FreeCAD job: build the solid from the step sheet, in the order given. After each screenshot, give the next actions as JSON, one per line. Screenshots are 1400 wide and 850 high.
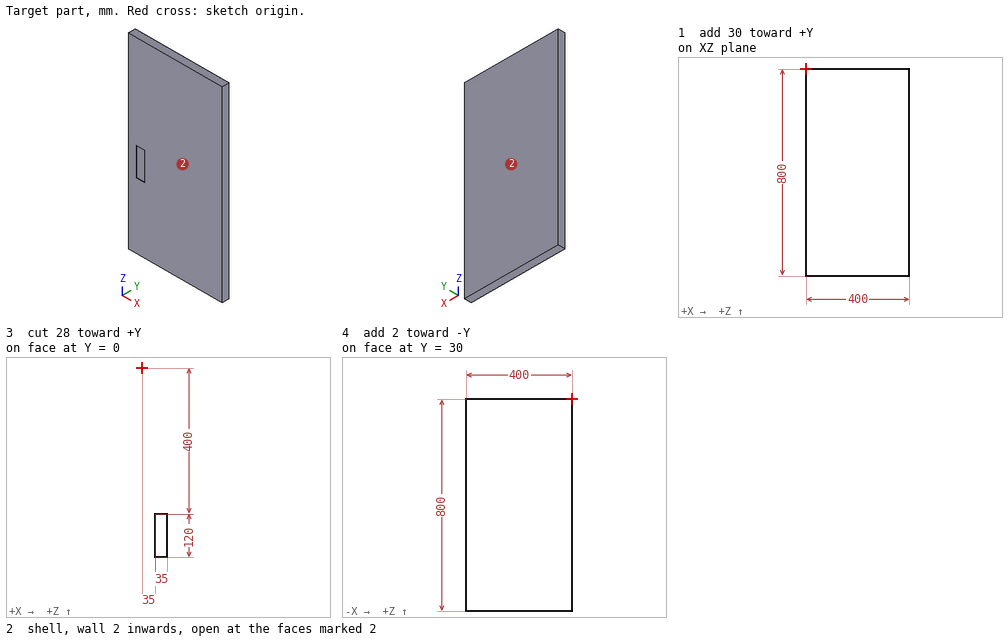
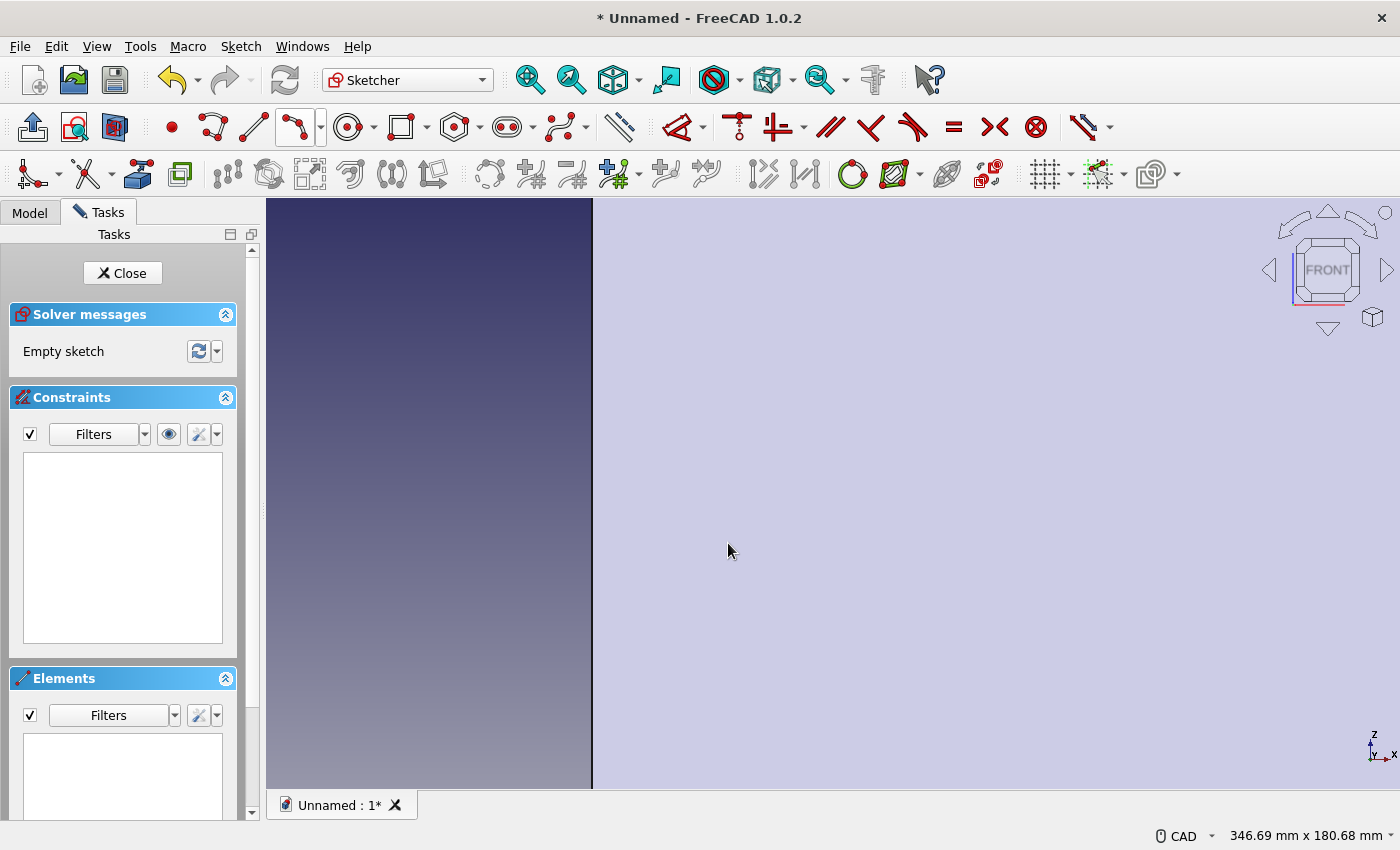
{"action": "left_click", "coordinate": [400, 128]}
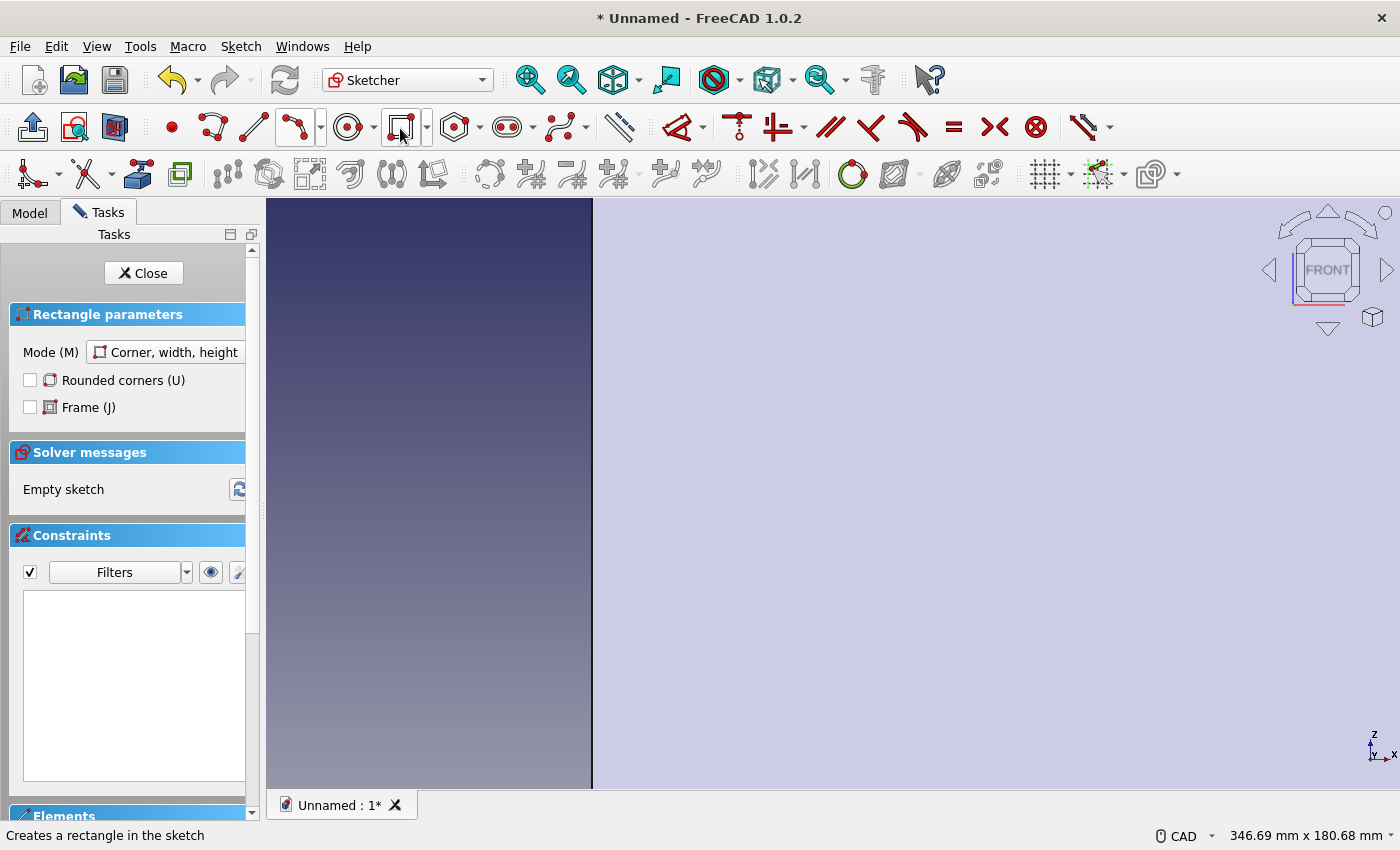
{"action": "left_click", "coordinate": [707, 296]}
{"action": "left_click", "coordinate": [821, 688]}
{"action": "key", "text": "Escape"}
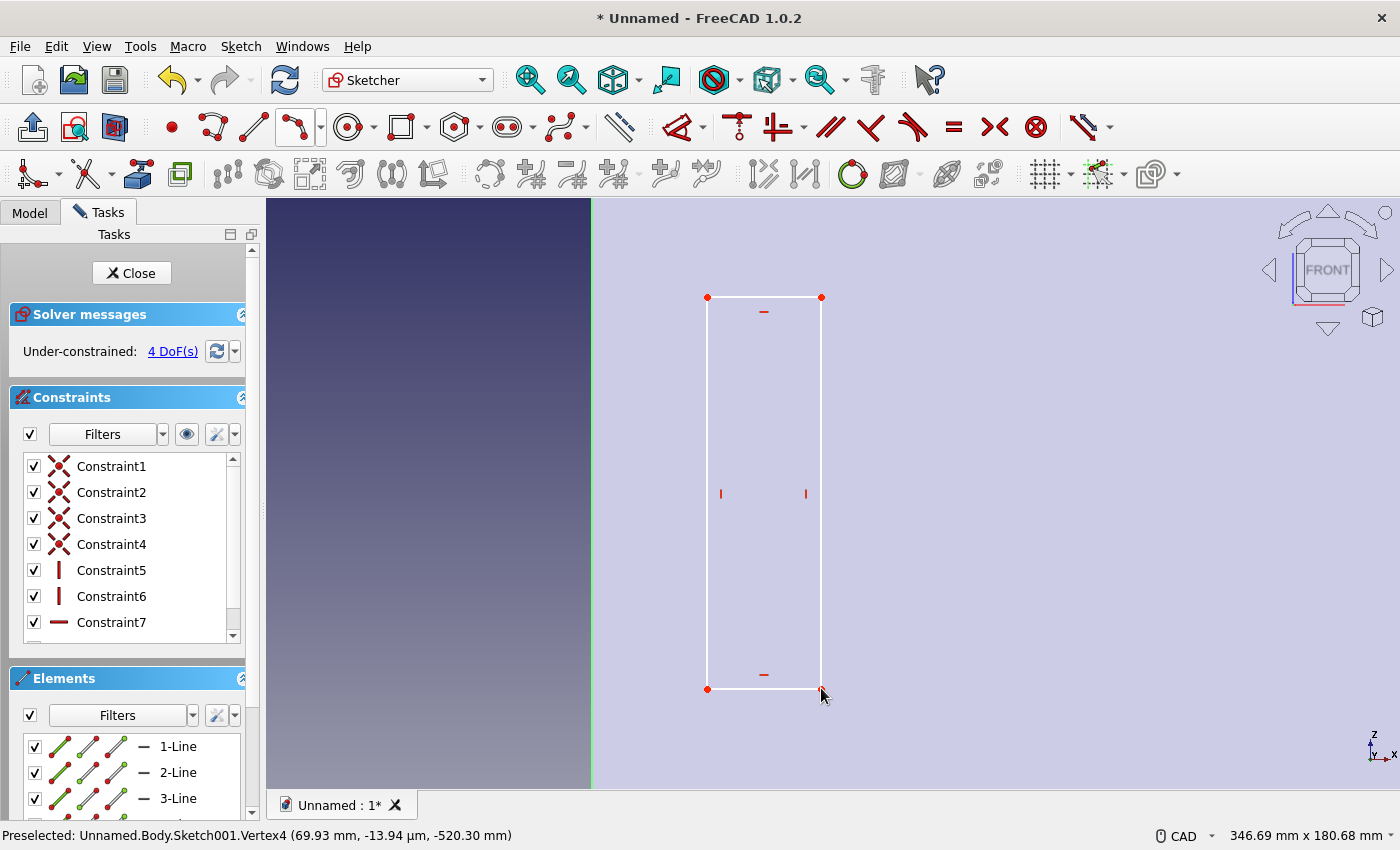
{"action": "left_click", "coordinate": [676, 128]}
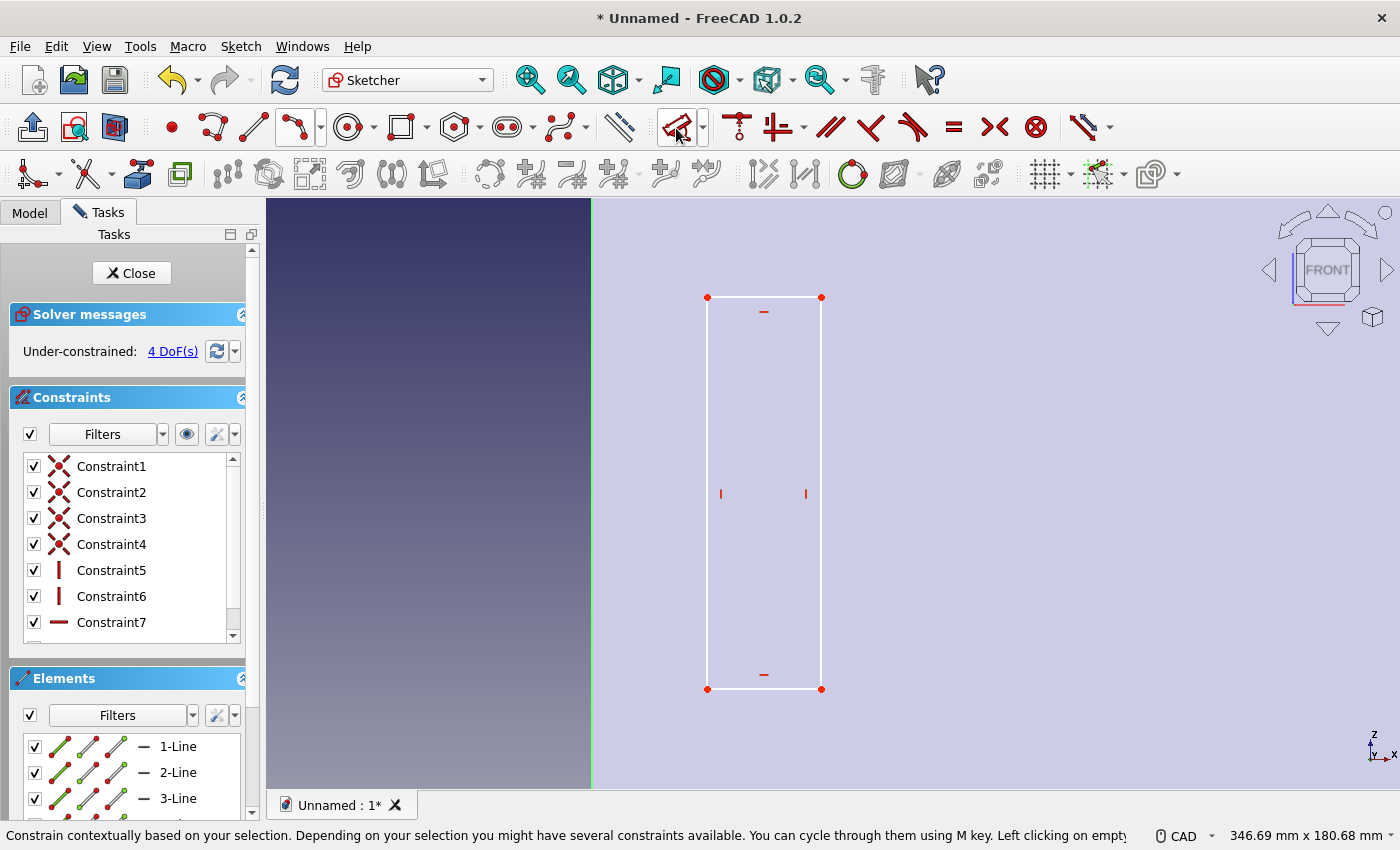
{"action": "left_click", "coordinate": [741, 689]}
{"action": "left_click", "coordinate": [764, 723]}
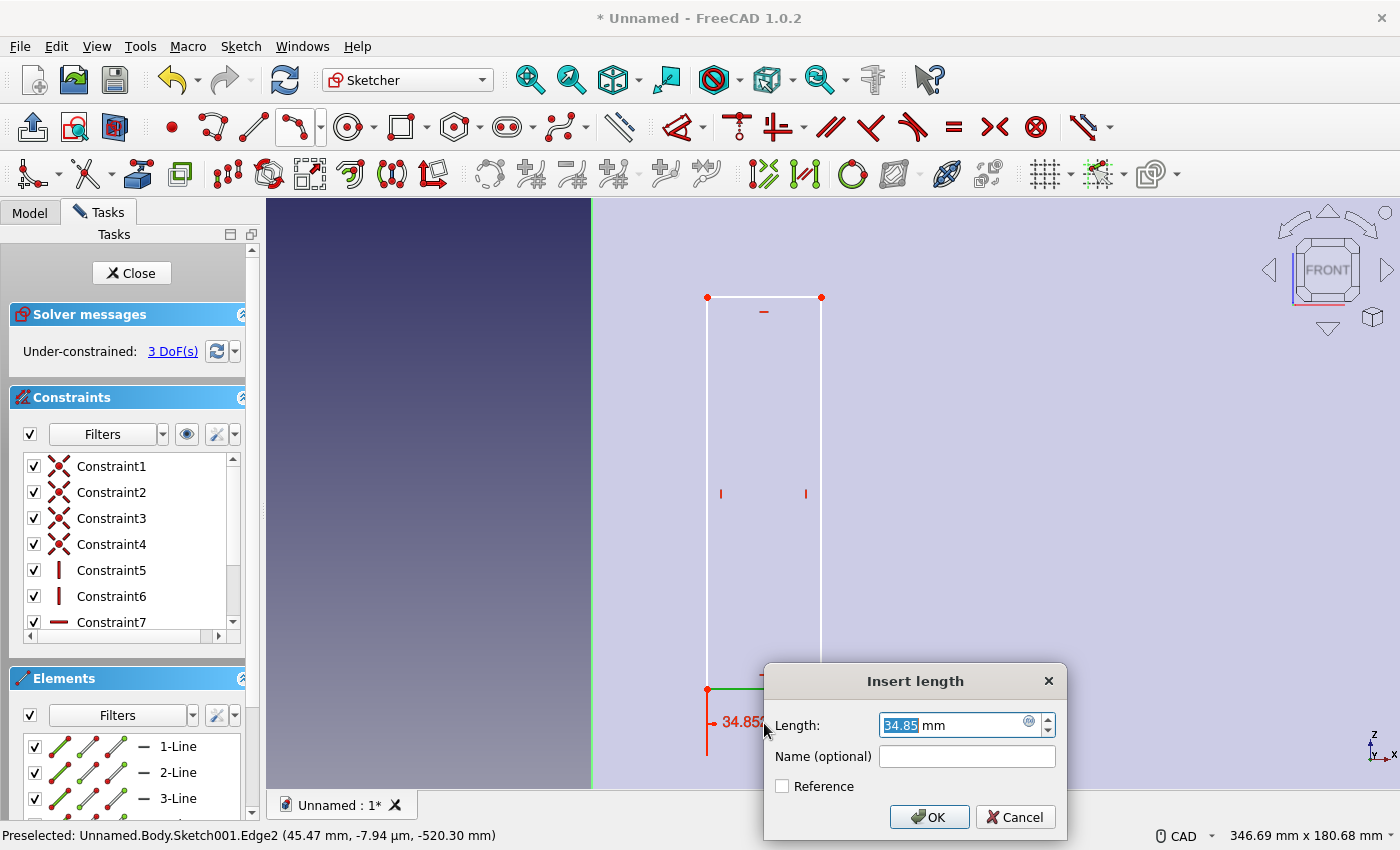
{"action": "type", "text": "35"}
{"action": "key", "text": "Return"}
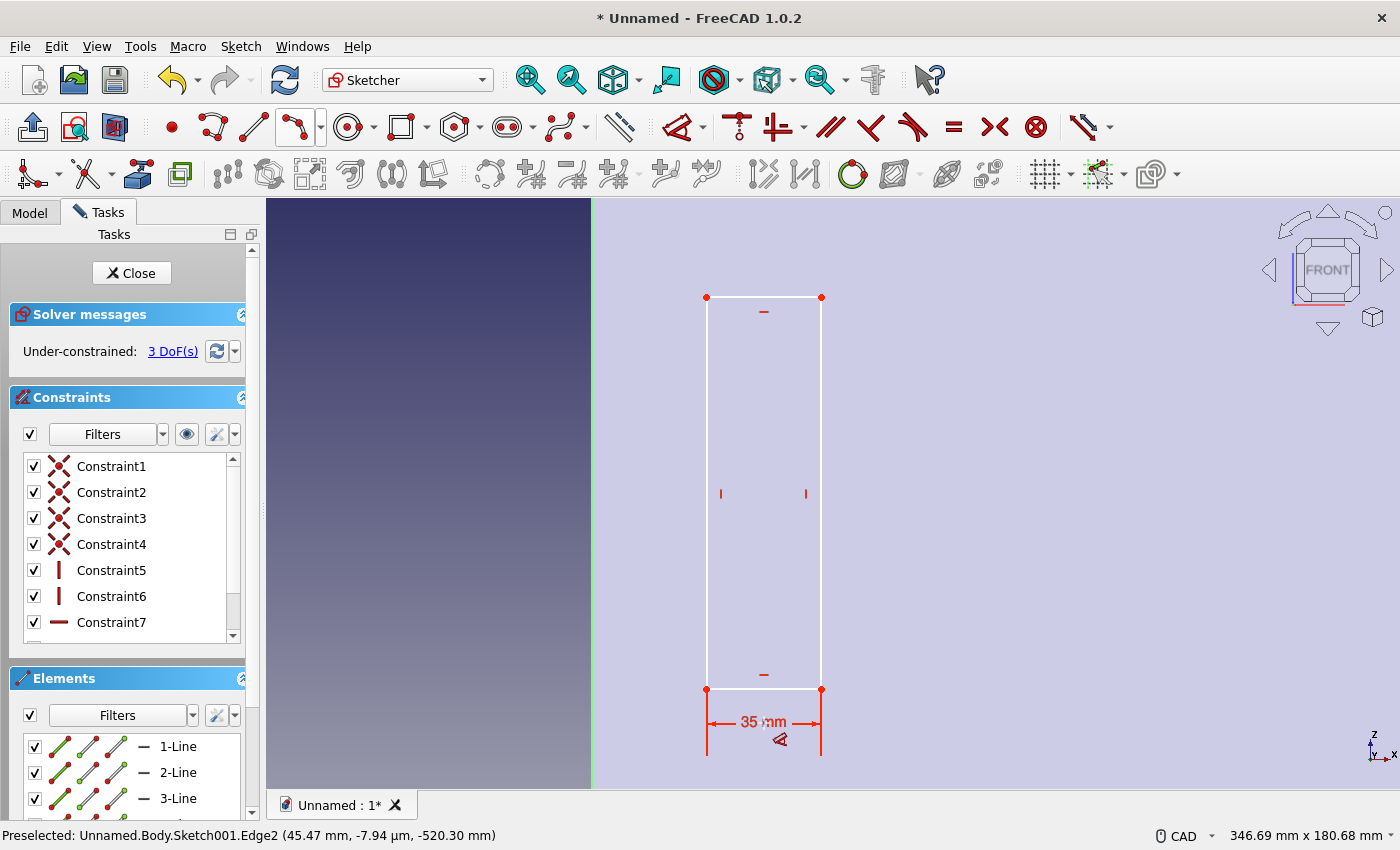
{"action": "left_click", "coordinate": [707, 415]}
{"action": "left_click", "coordinate": [673, 493]}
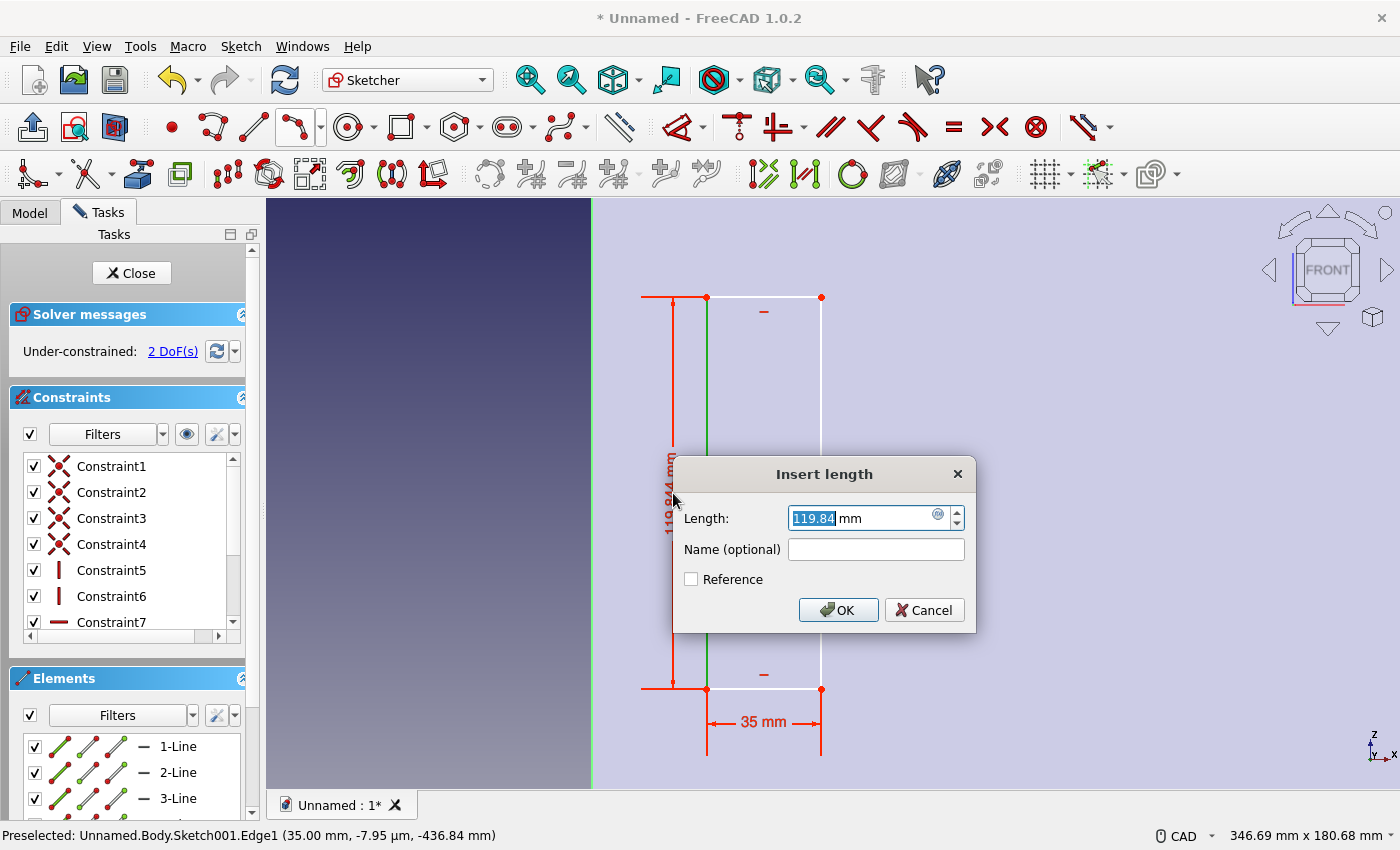
{"action": "type", "text": "120"}
{"action": "key", "text": "Return"}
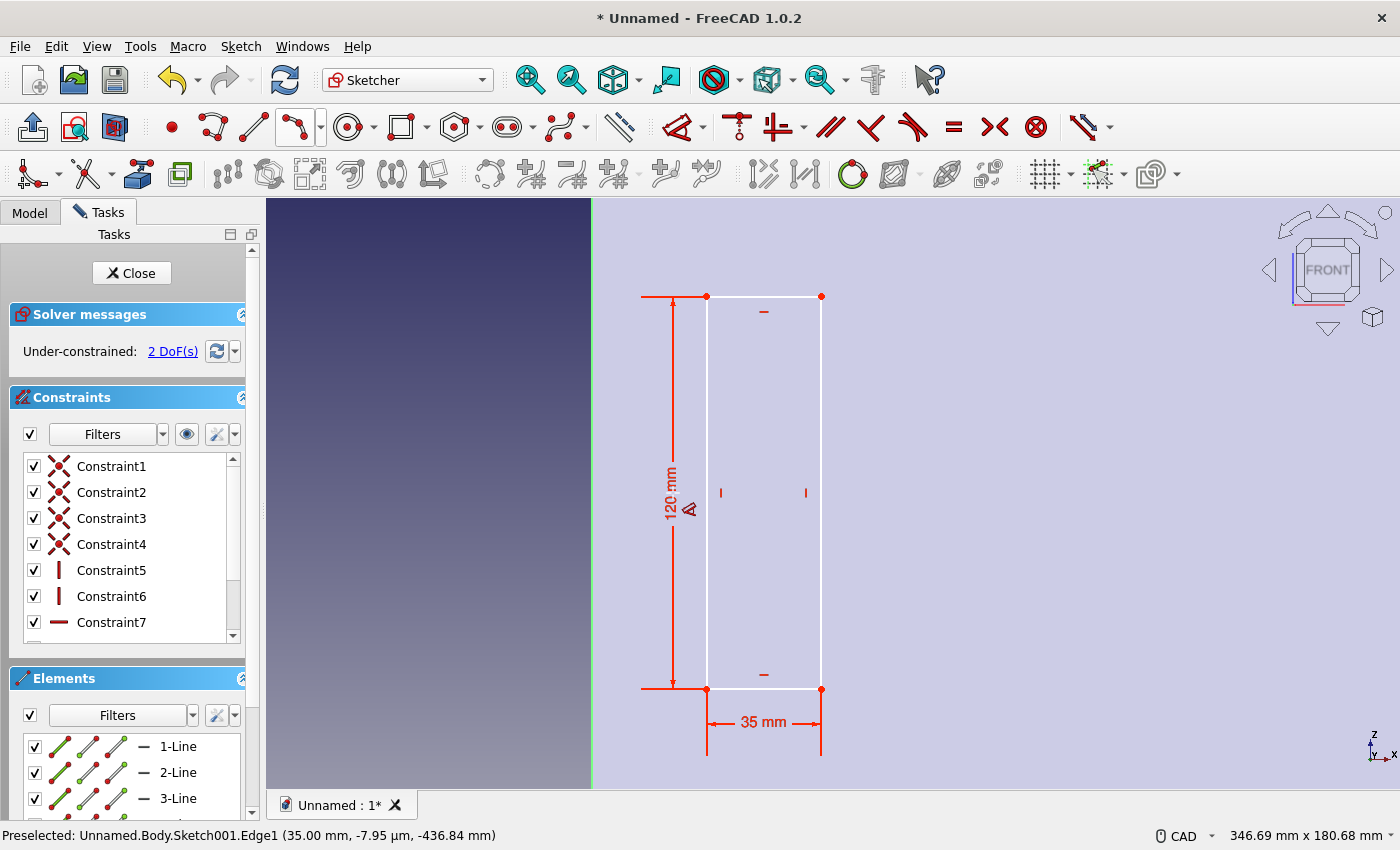
{"action": "left_click", "coordinate": [707, 297]}
{"action": "left_click", "coordinate": [650, 331]}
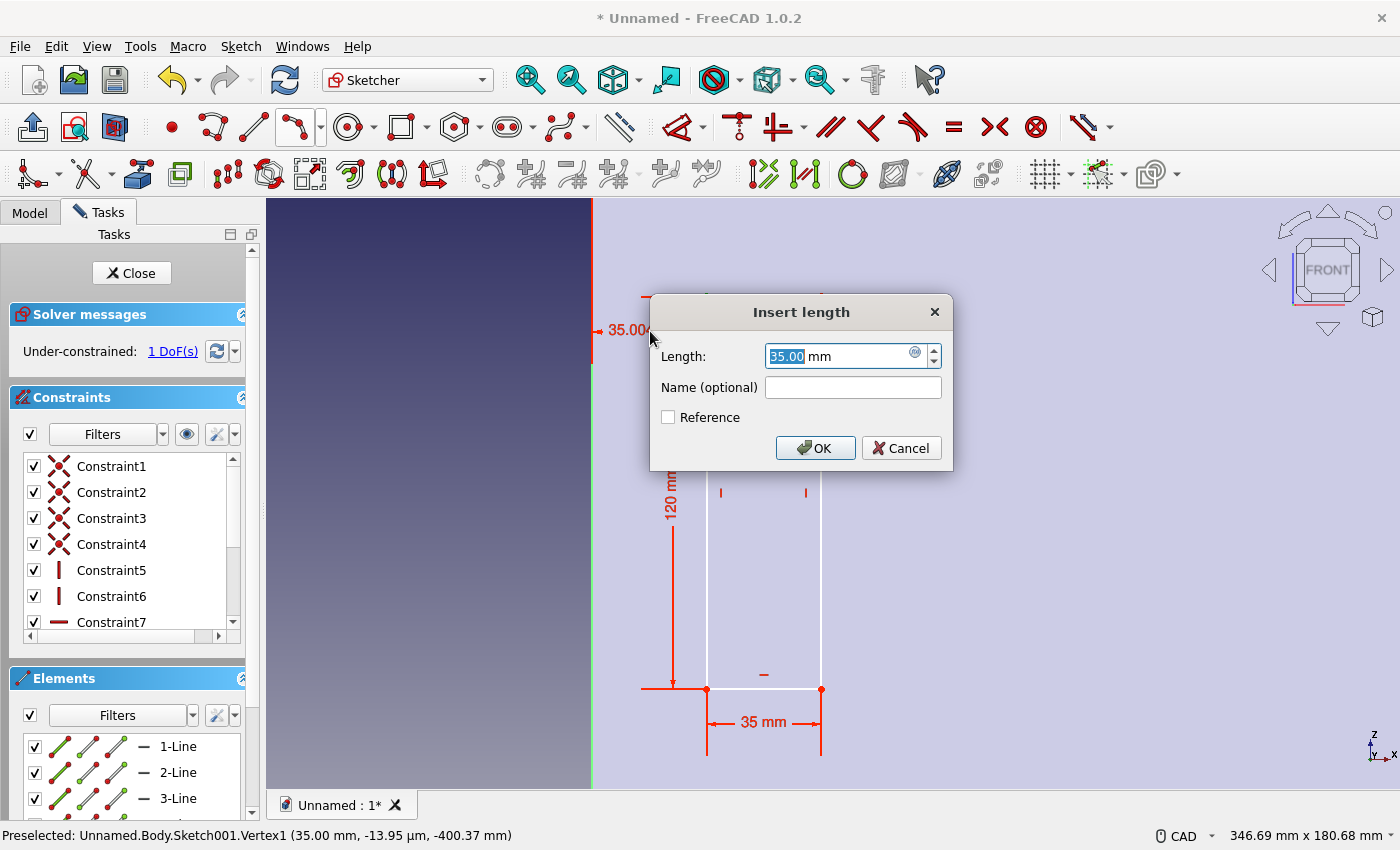
{"action": "type", "text": "35"}
{"action": "key", "text": "Return"}